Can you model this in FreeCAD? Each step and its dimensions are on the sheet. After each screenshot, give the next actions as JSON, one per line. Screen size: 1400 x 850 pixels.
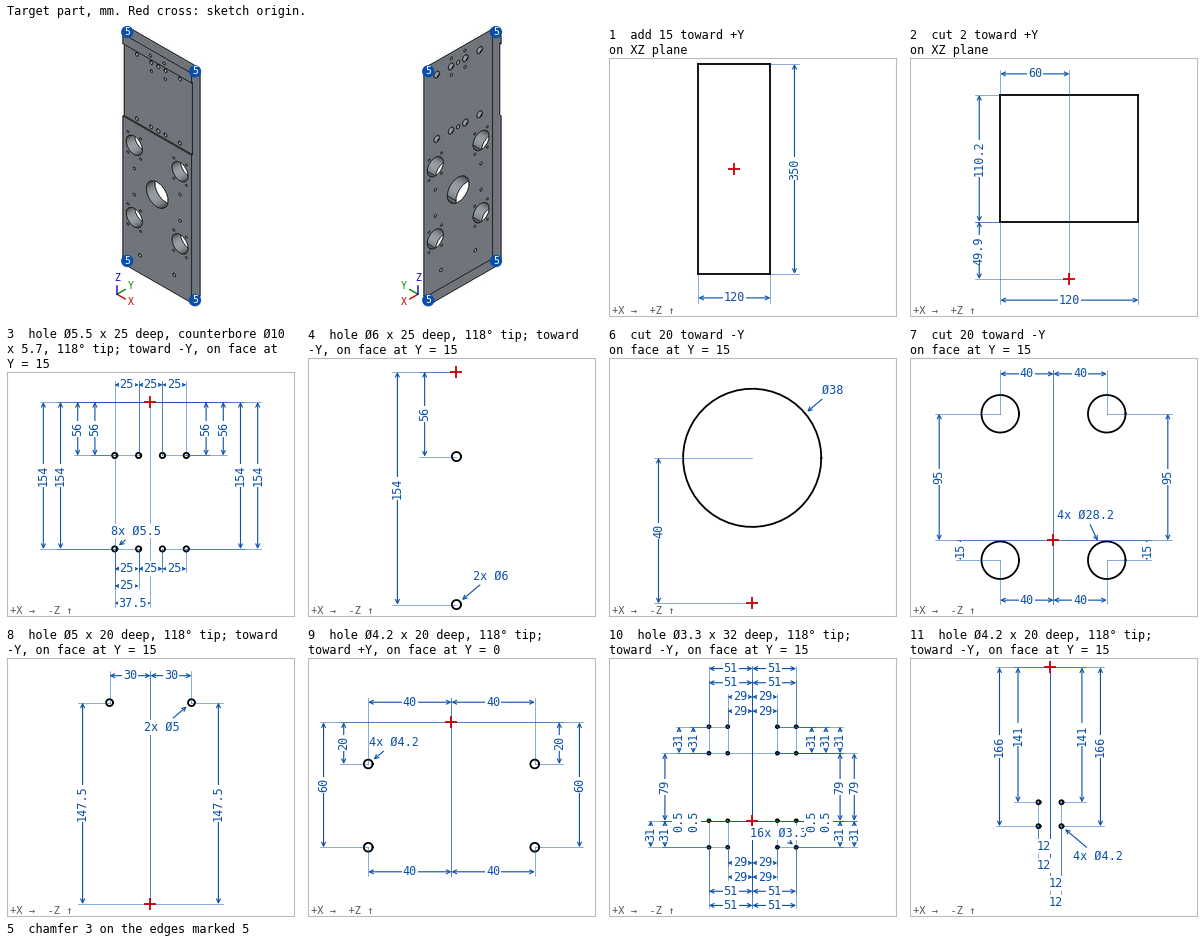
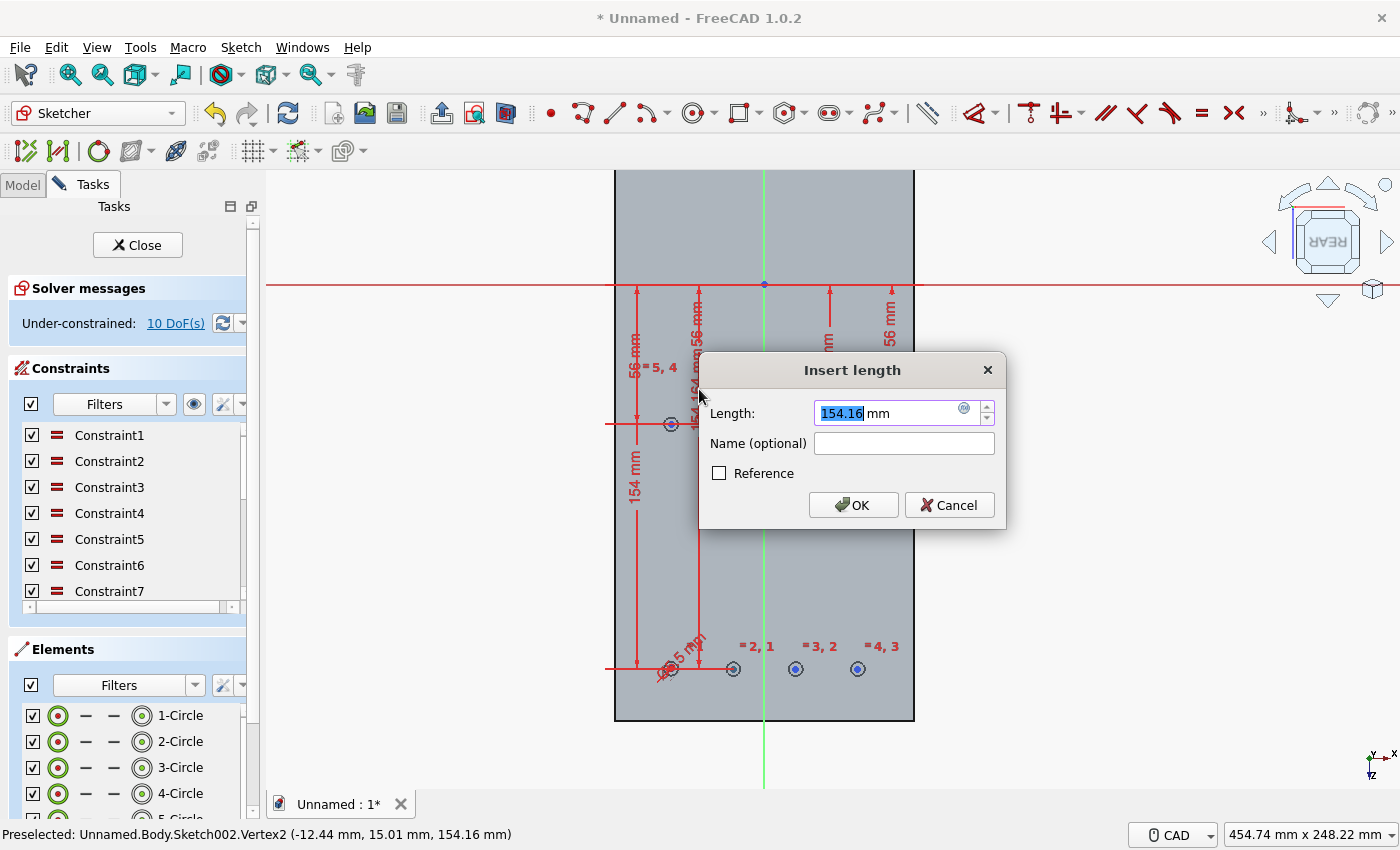
{"action": "type", "text": "154"}
{"action": "key", "text": "Return"}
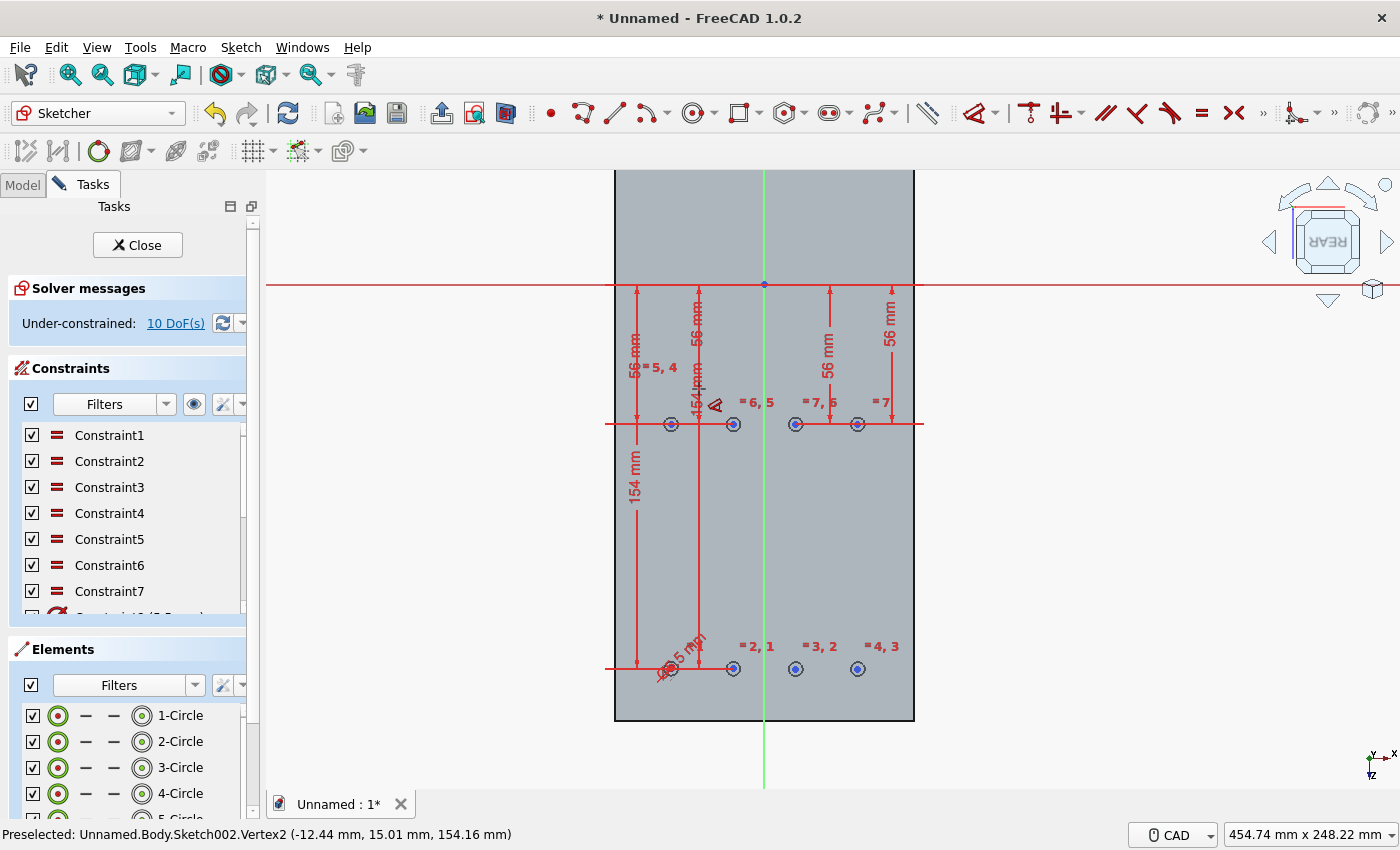
{"action": "left_click", "coordinate": [796, 669]}
{"action": "left_click", "coordinate": [830, 477]}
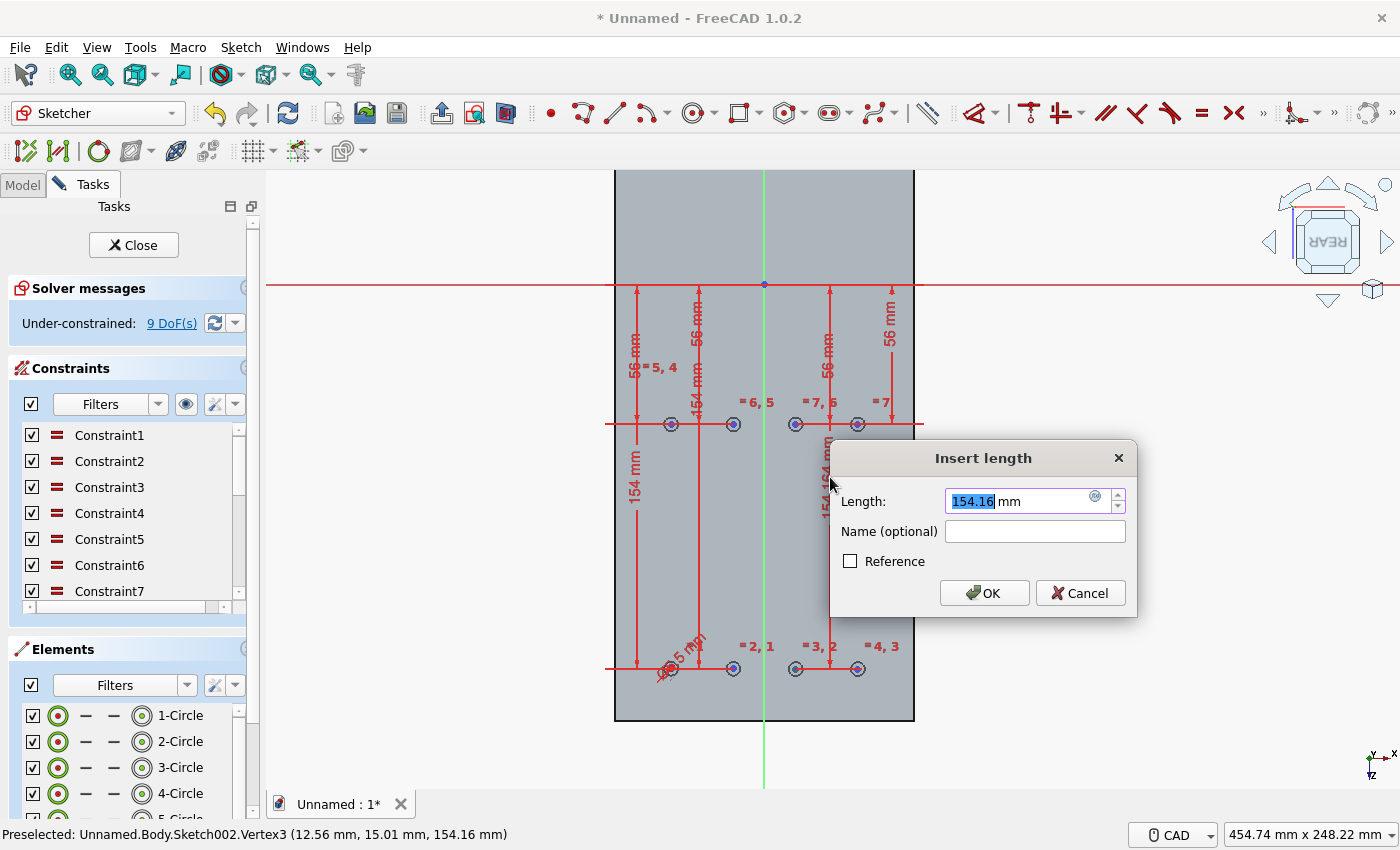
{"action": "type", "text": "154"}
{"action": "key", "text": "Return"}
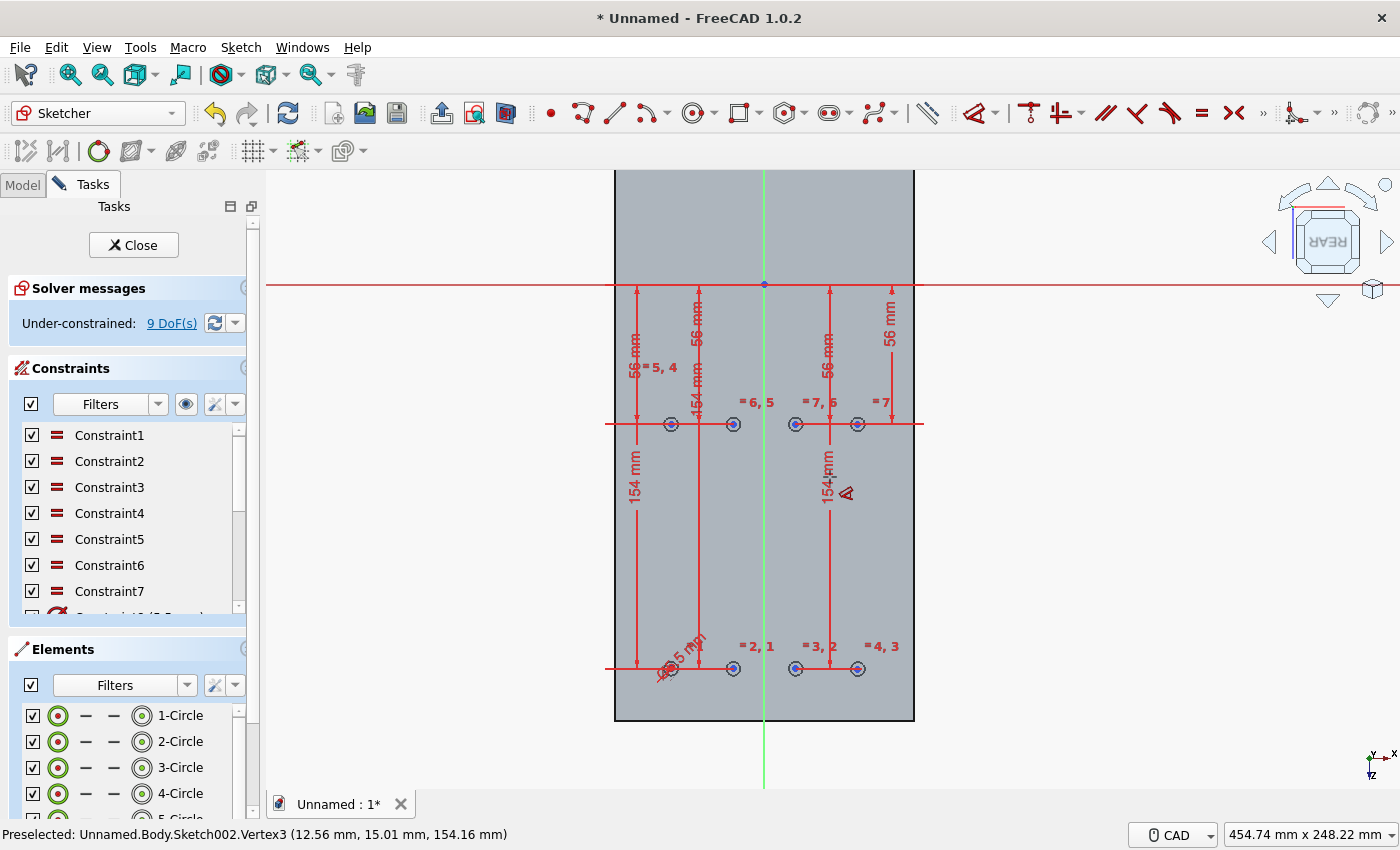
{"action": "left_click", "coordinate": [858, 669]}
{"action": "left_click", "coordinate": [892, 389]}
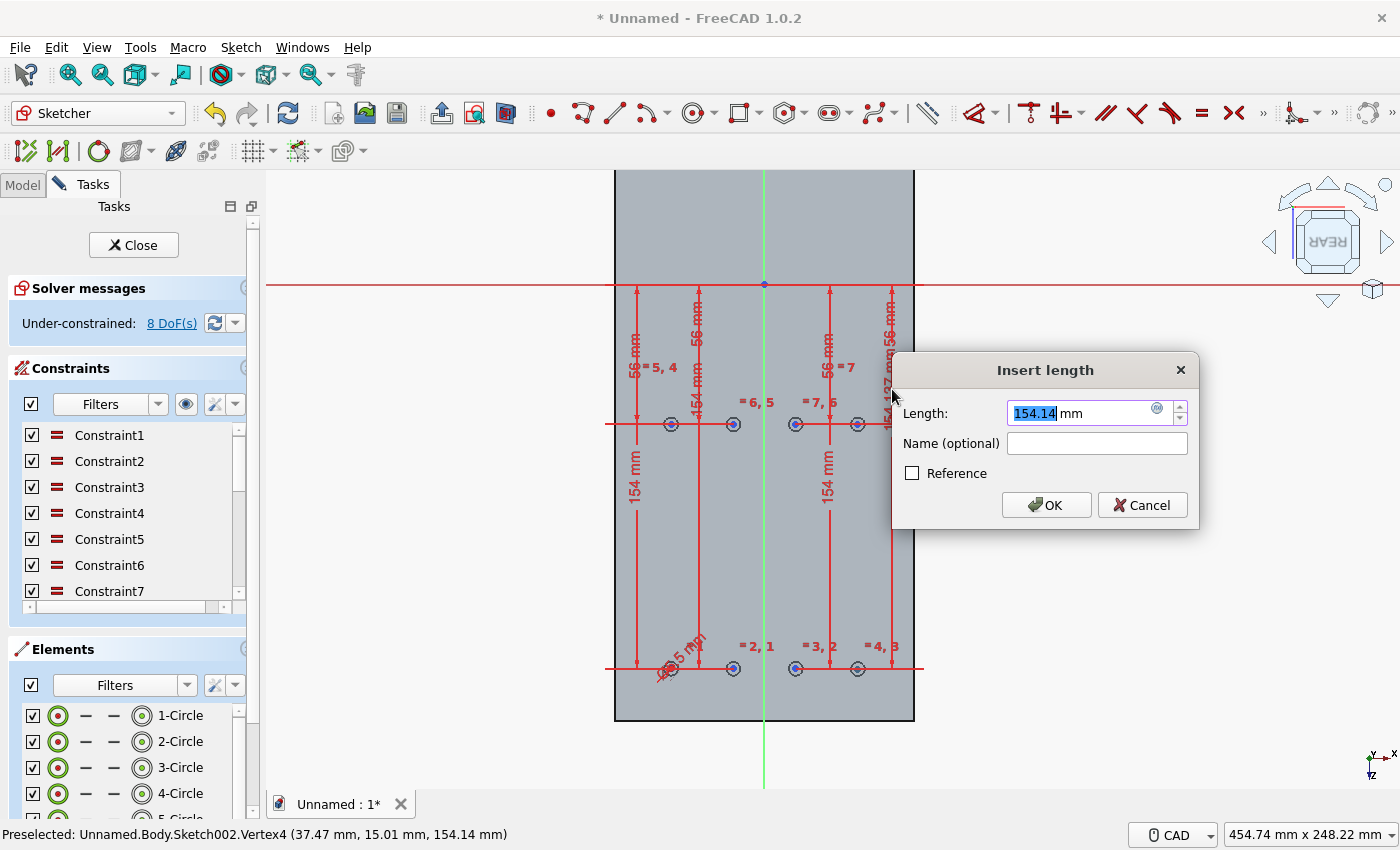
{"action": "type", "text": "154"}
{"action": "key", "text": "Return"}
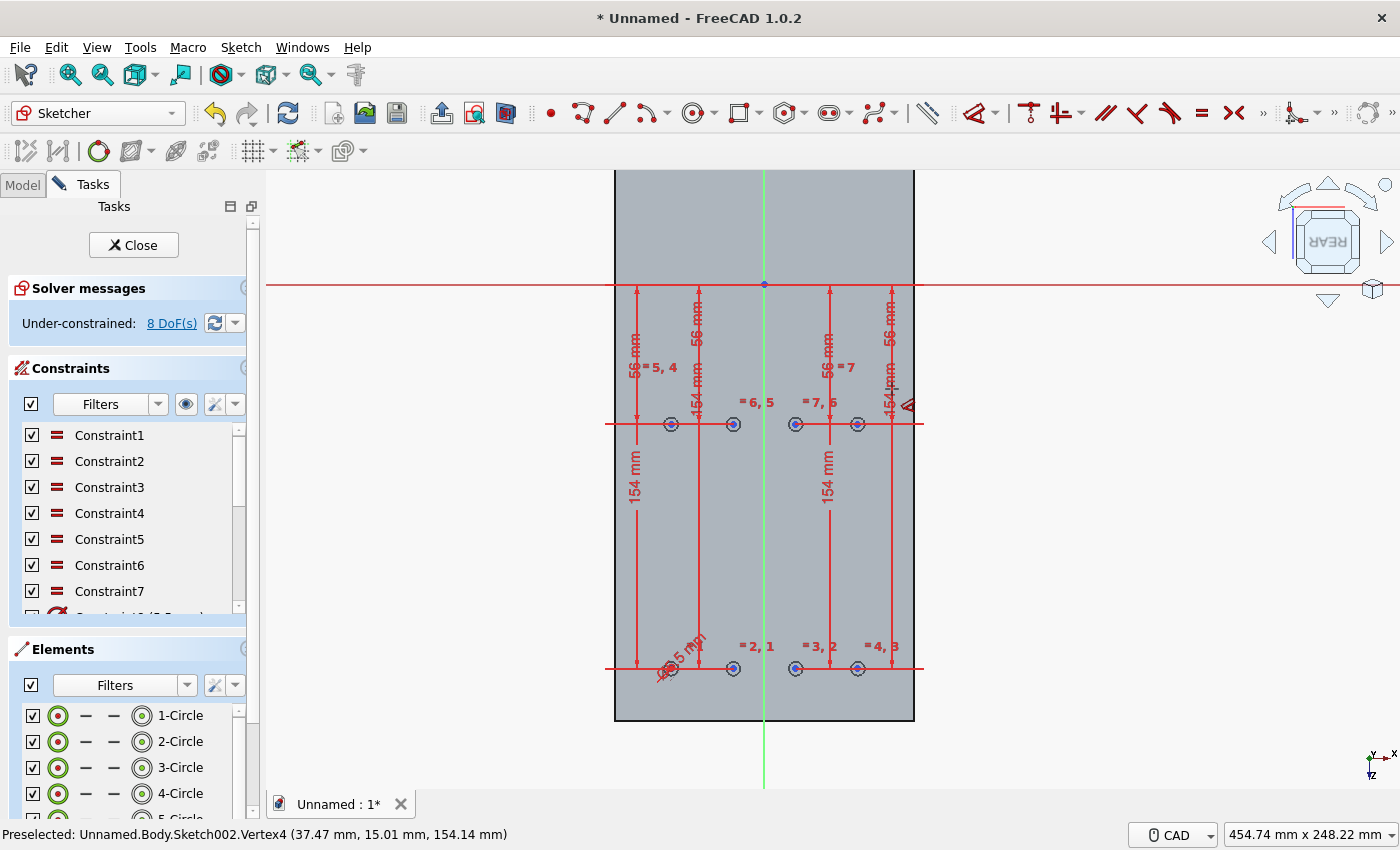
{"action": "left_click", "coordinate": [671, 669]}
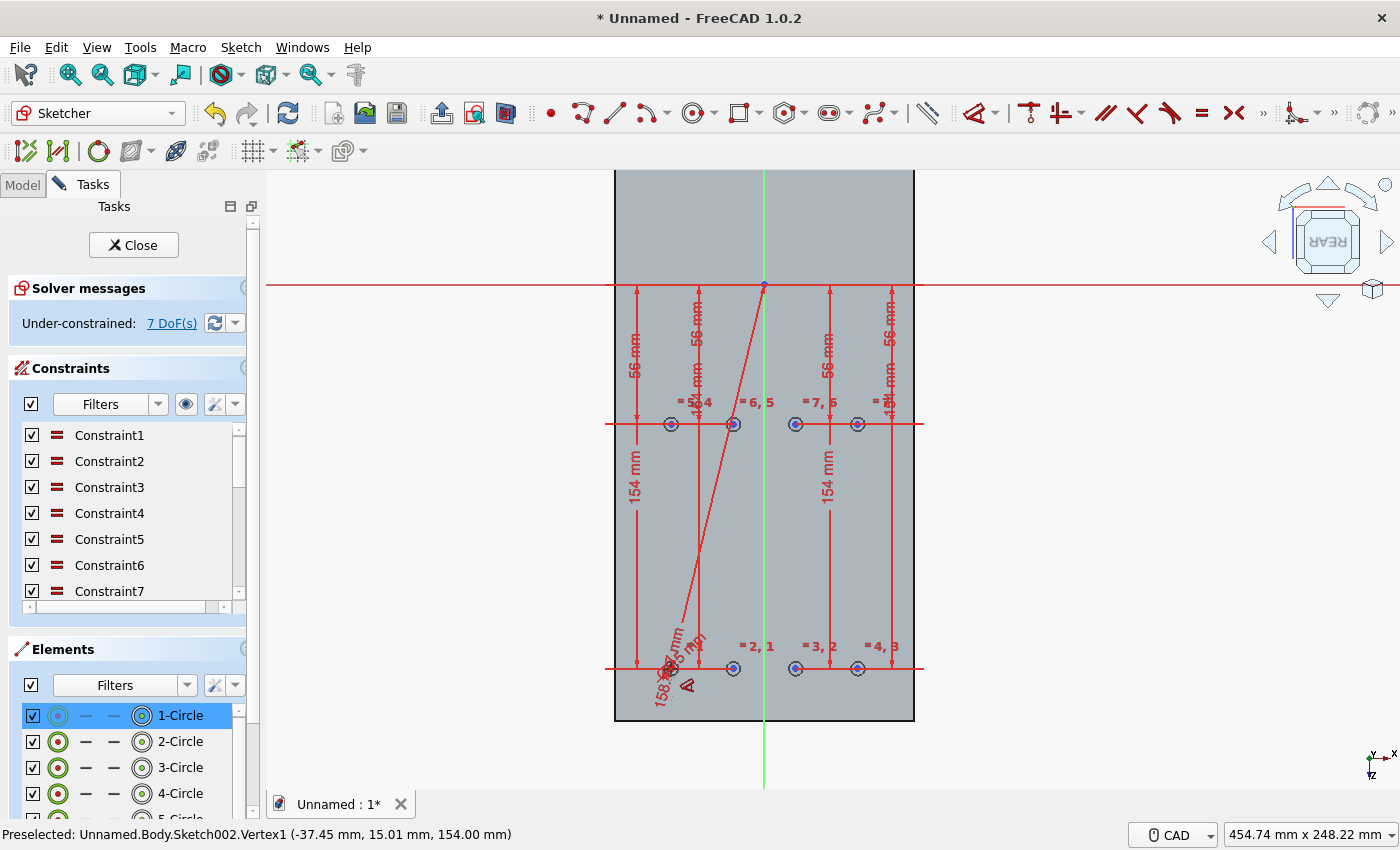
{"action": "left_click", "coordinate": [733, 669]}
{"action": "left_click", "coordinate": [702, 703]}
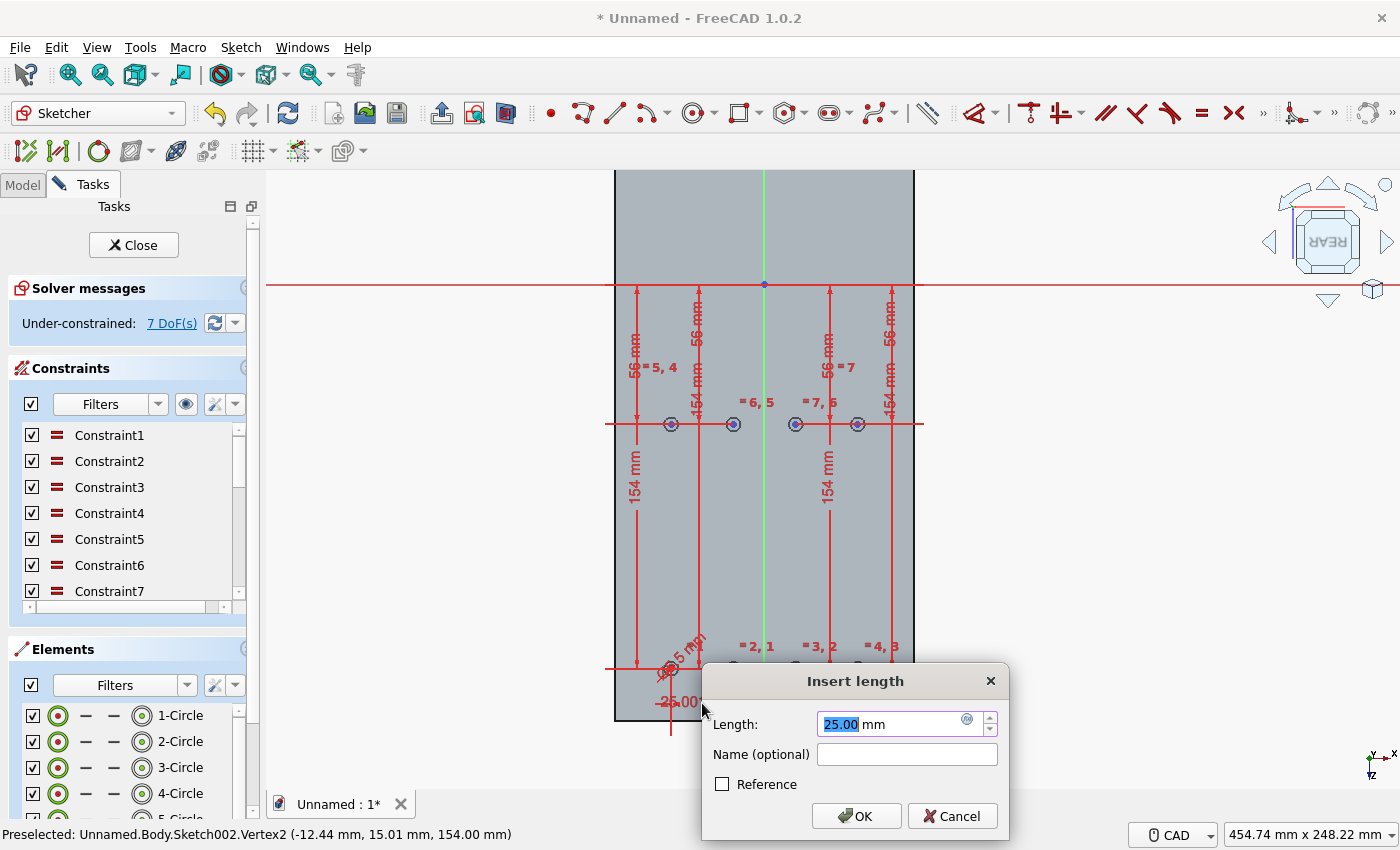
{"action": "type", "text": "25"}
{"action": "key", "text": "Return"}